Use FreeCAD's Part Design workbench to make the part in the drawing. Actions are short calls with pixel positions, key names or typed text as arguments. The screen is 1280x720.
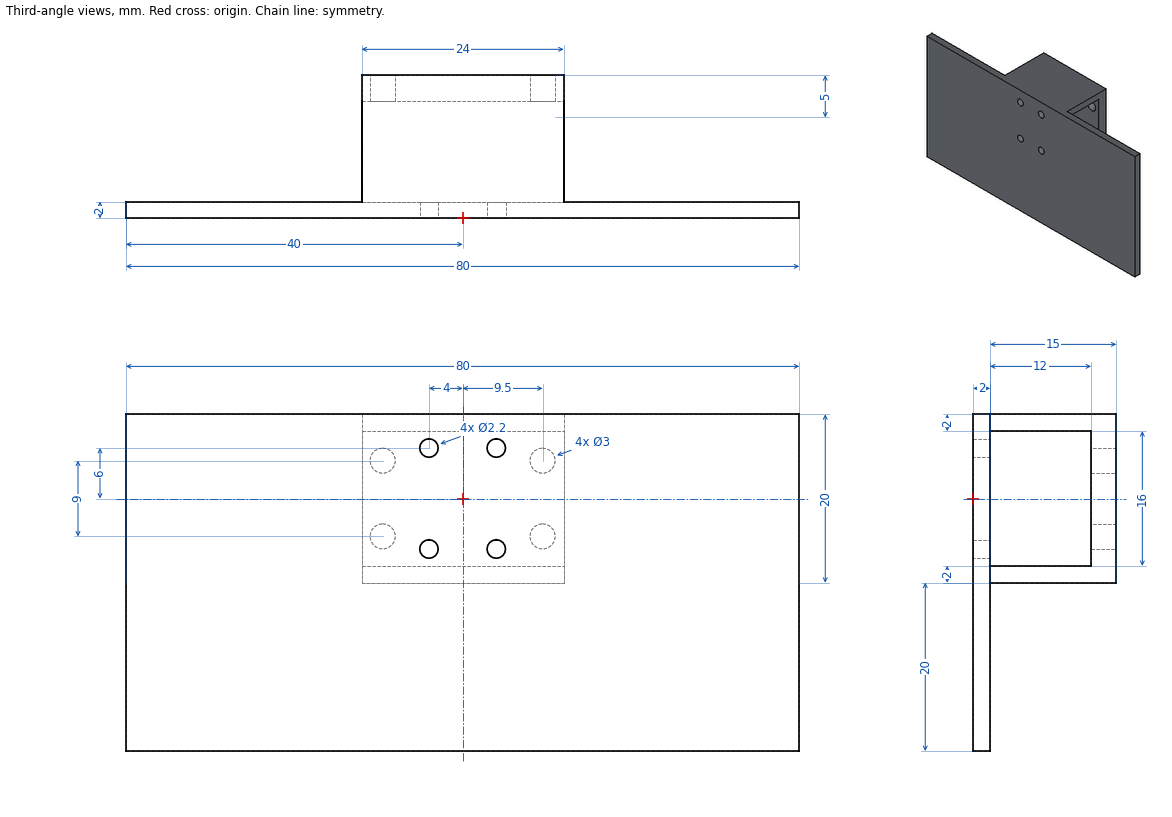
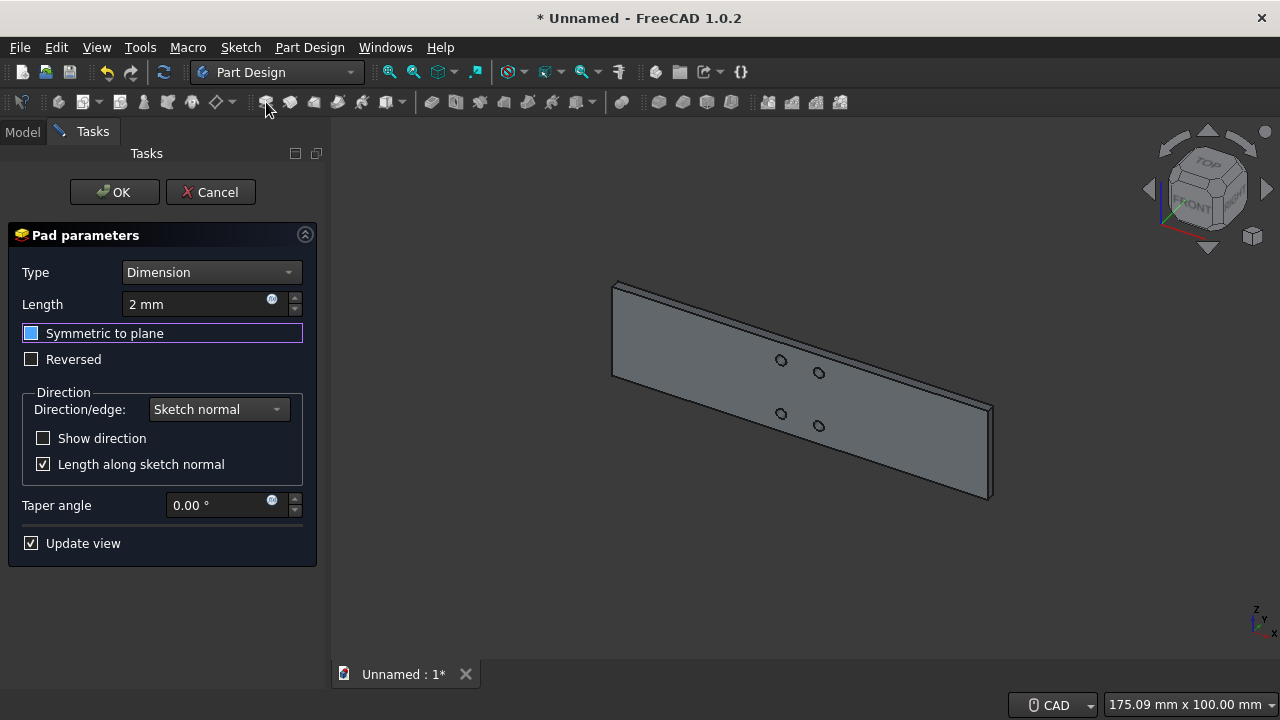
click(30, 359)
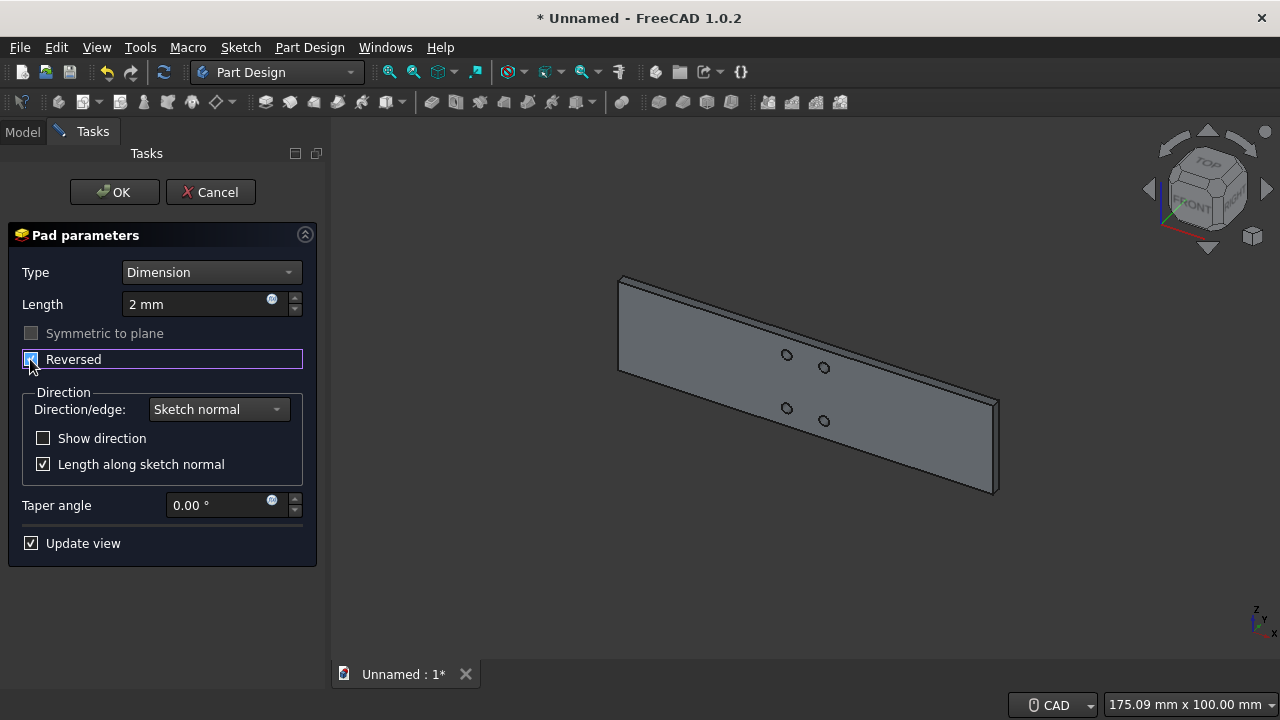
click(115, 192)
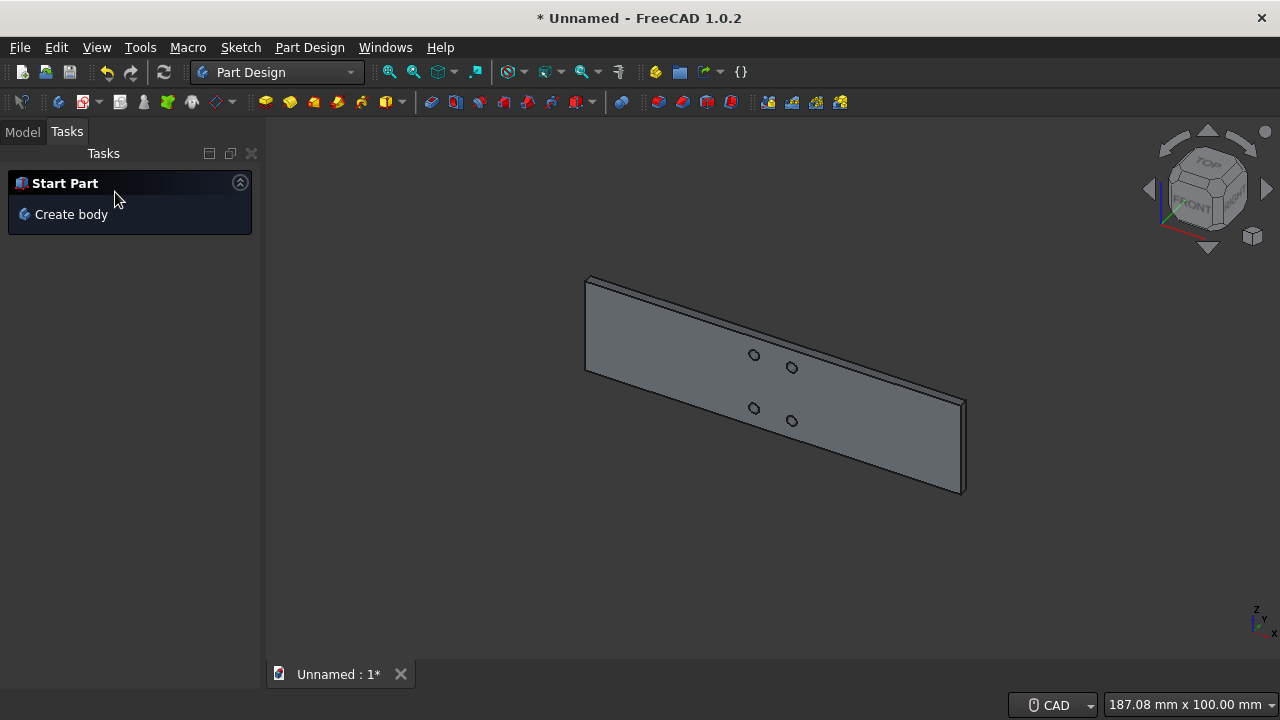
click(390, 72)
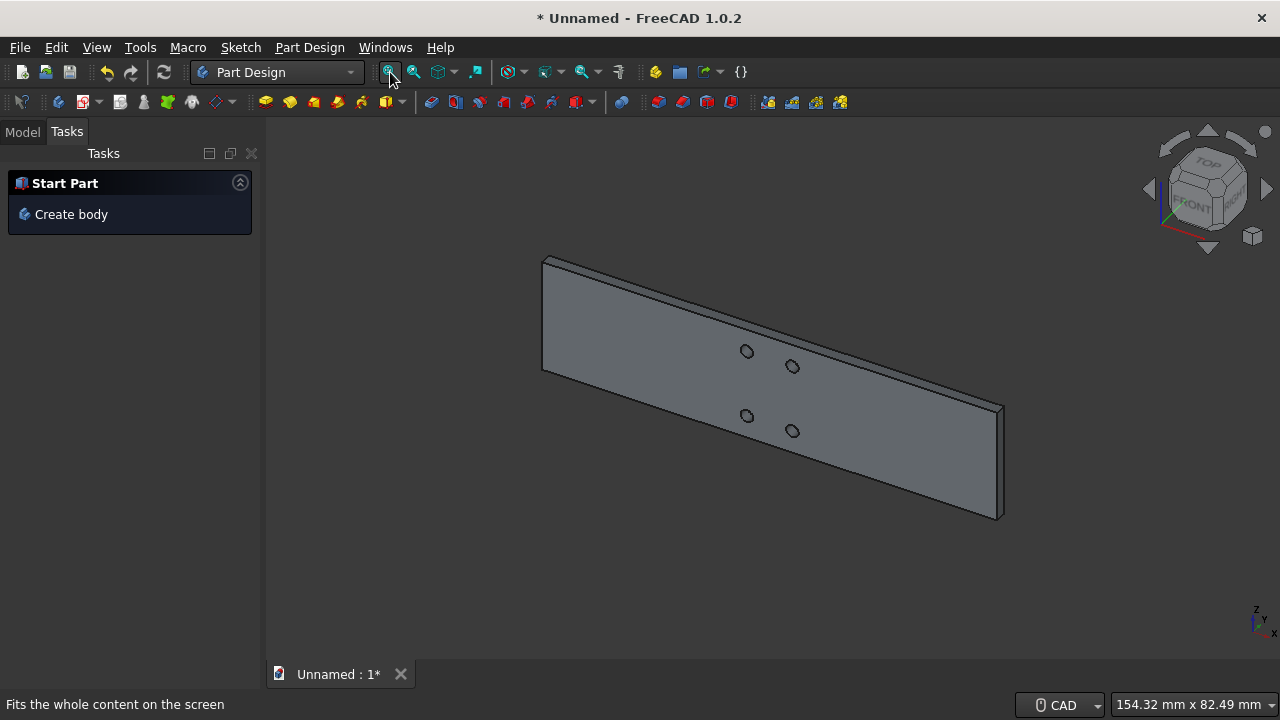
click(84, 102)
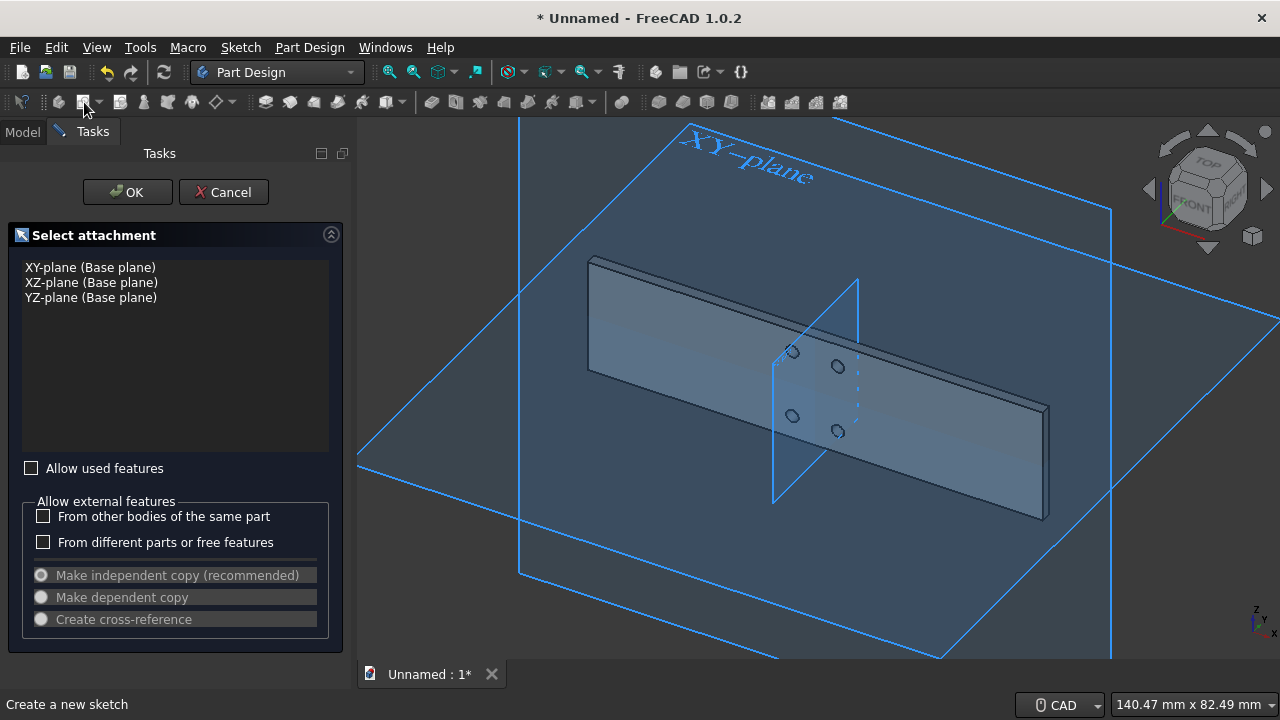
click(82, 298)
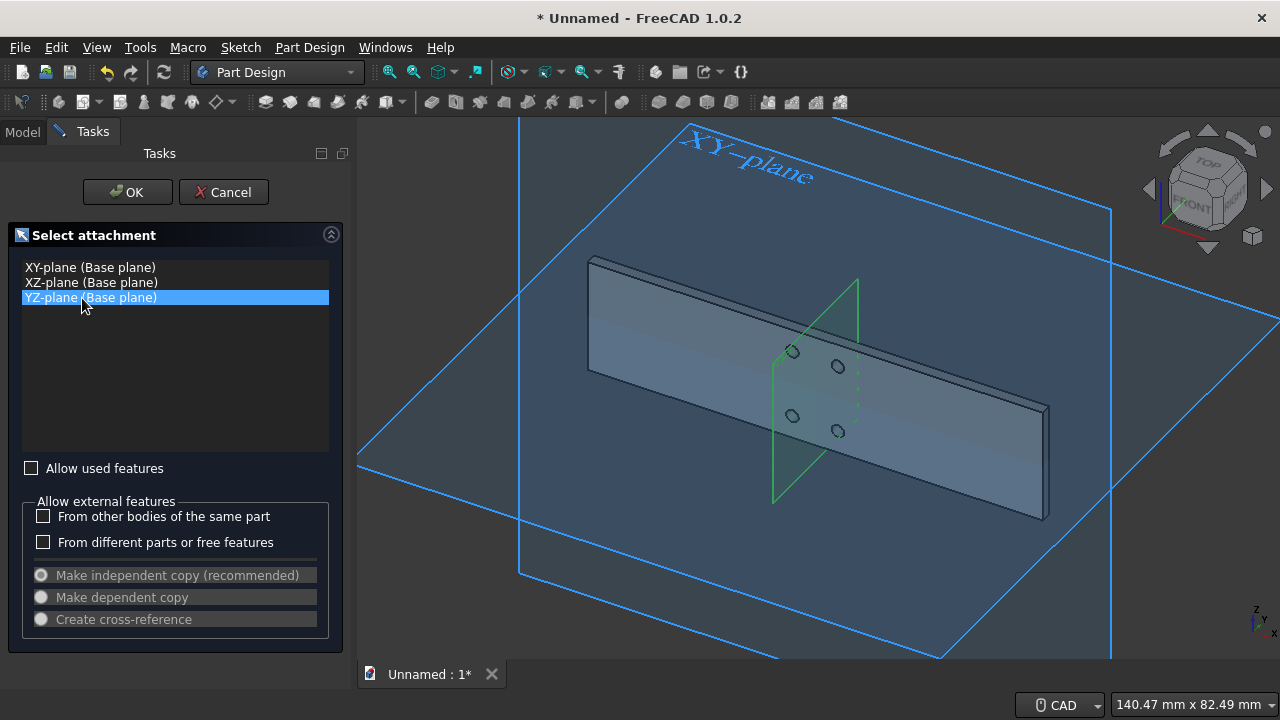
click(128, 192)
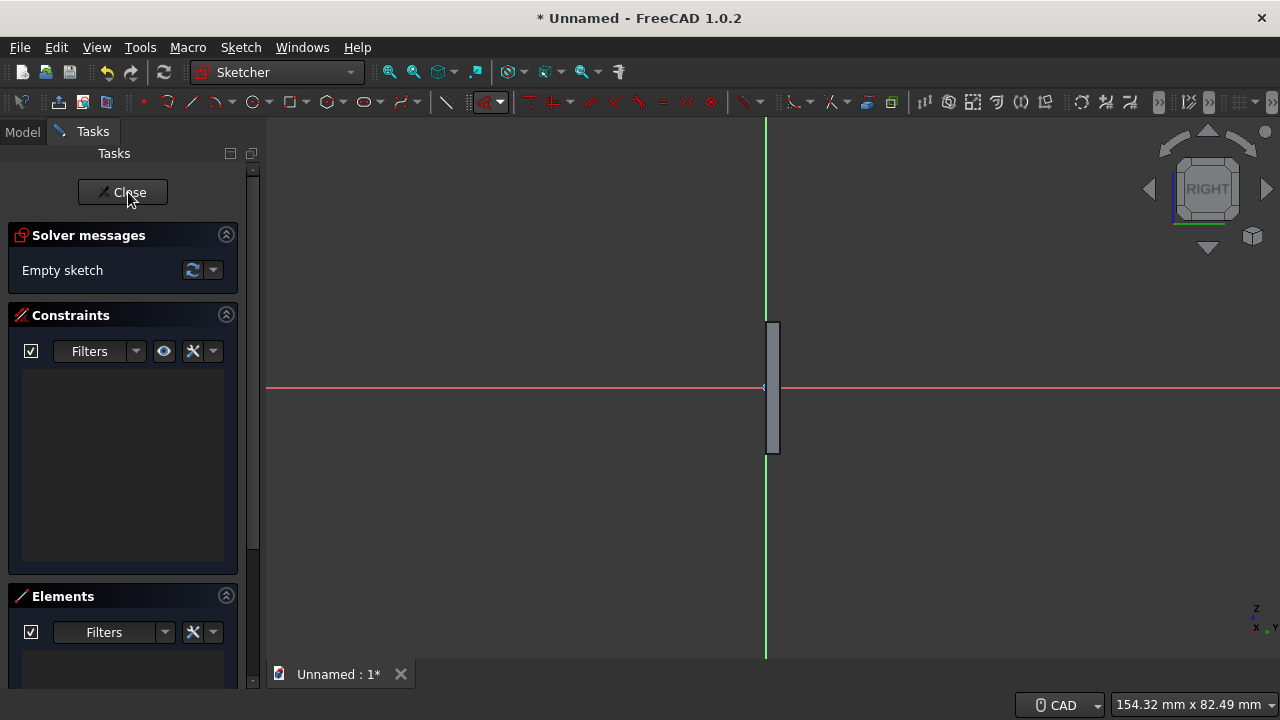
click(108, 102)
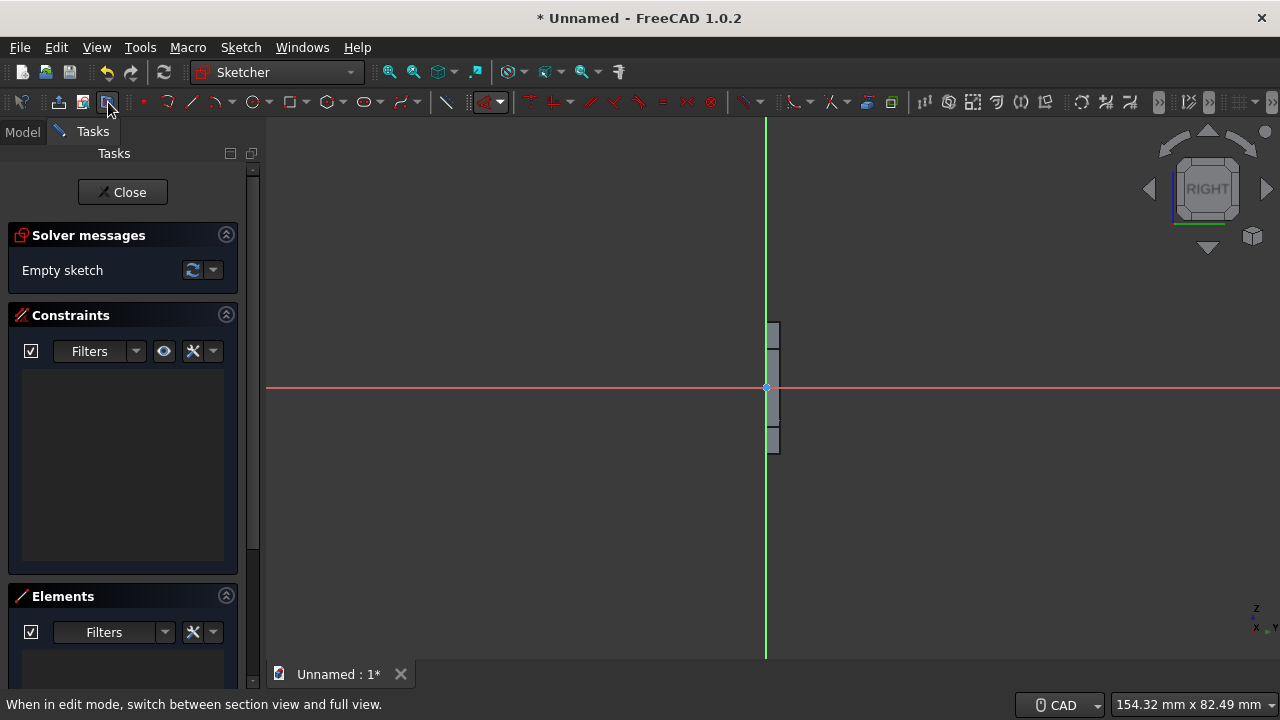
scroll(891, 388, up, 5)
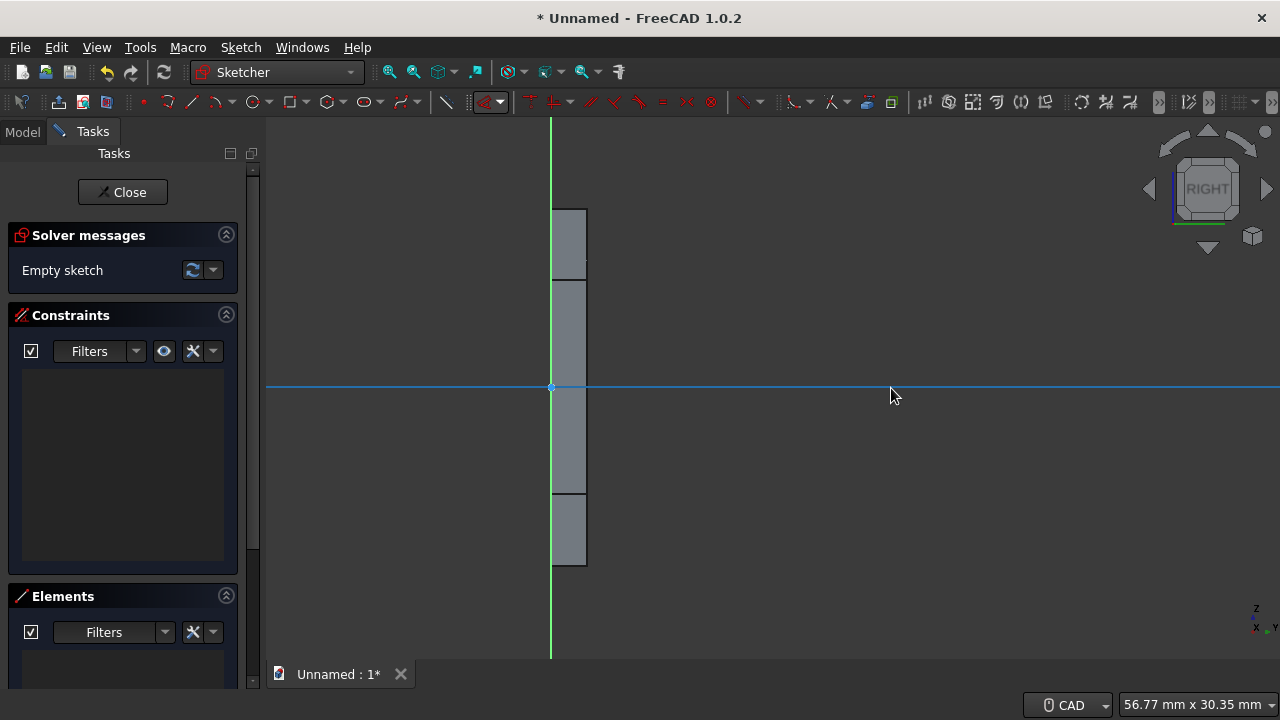
click(168, 102)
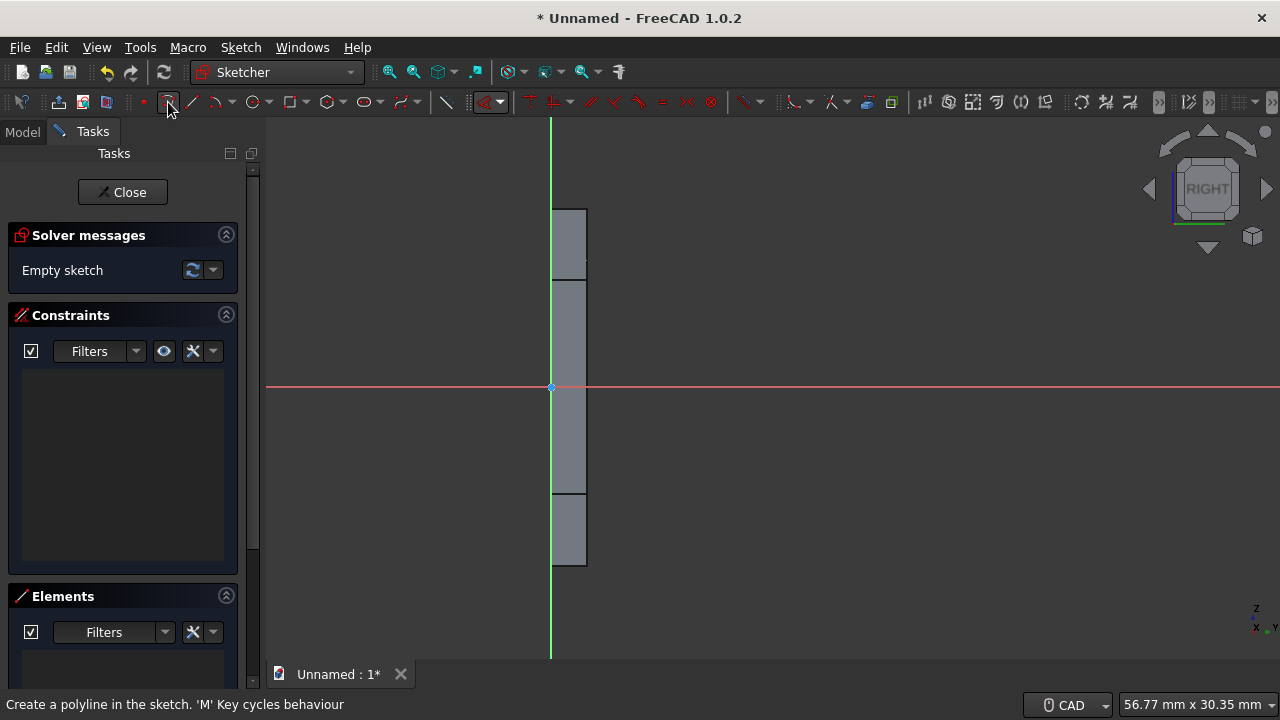
click(587, 244)
click(801, 244)
click(801, 530)
click(587, 530)
click(587, 566)
click(855, 566)
click(855, 209)
click(587, 209)
click(587, 245)
key(Escape)
key(Escape)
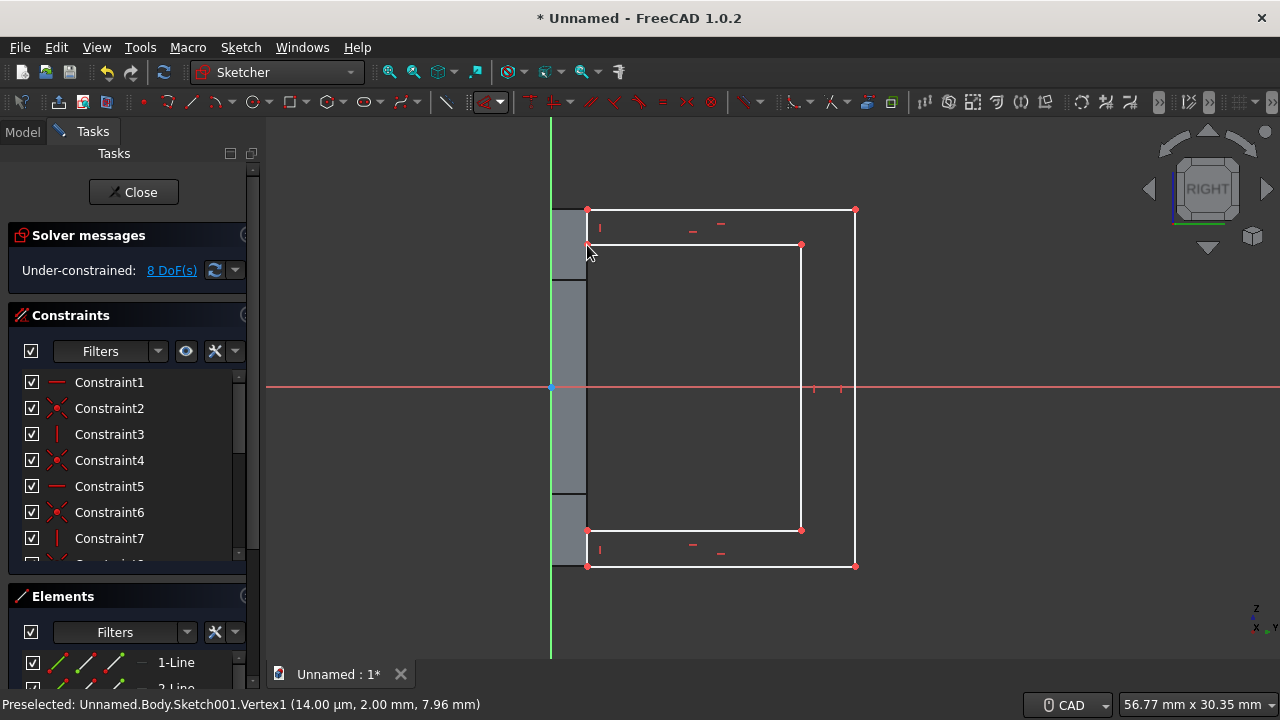
click(587, 245)